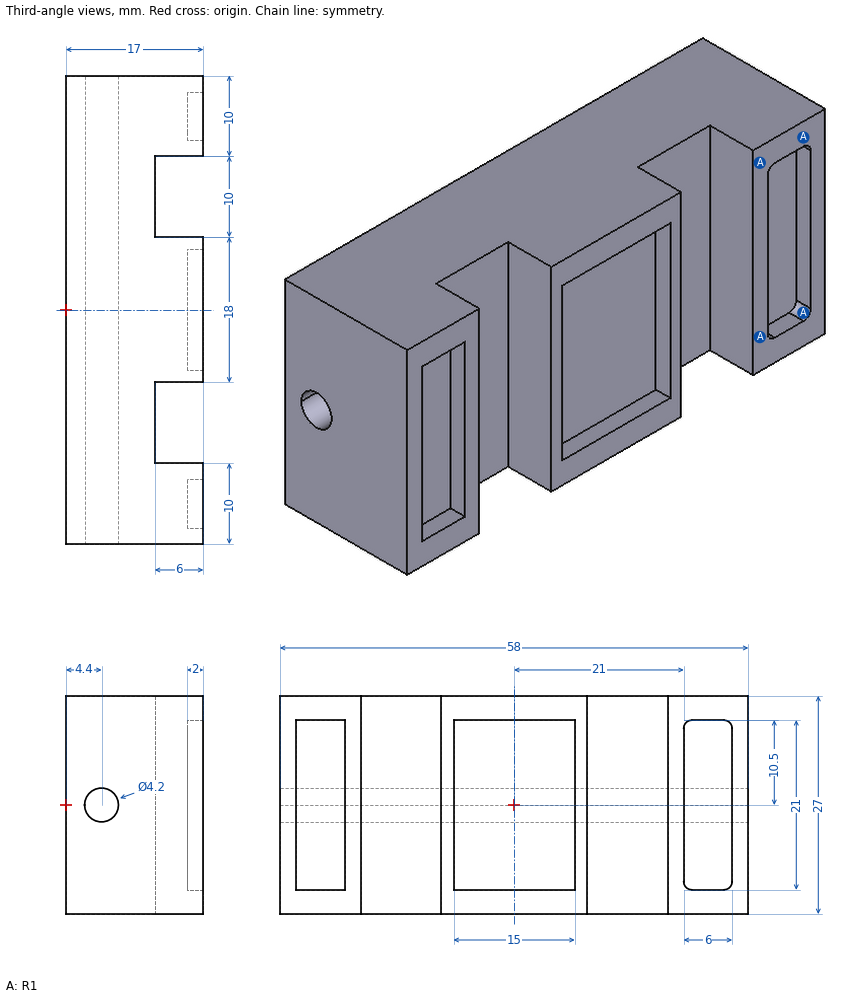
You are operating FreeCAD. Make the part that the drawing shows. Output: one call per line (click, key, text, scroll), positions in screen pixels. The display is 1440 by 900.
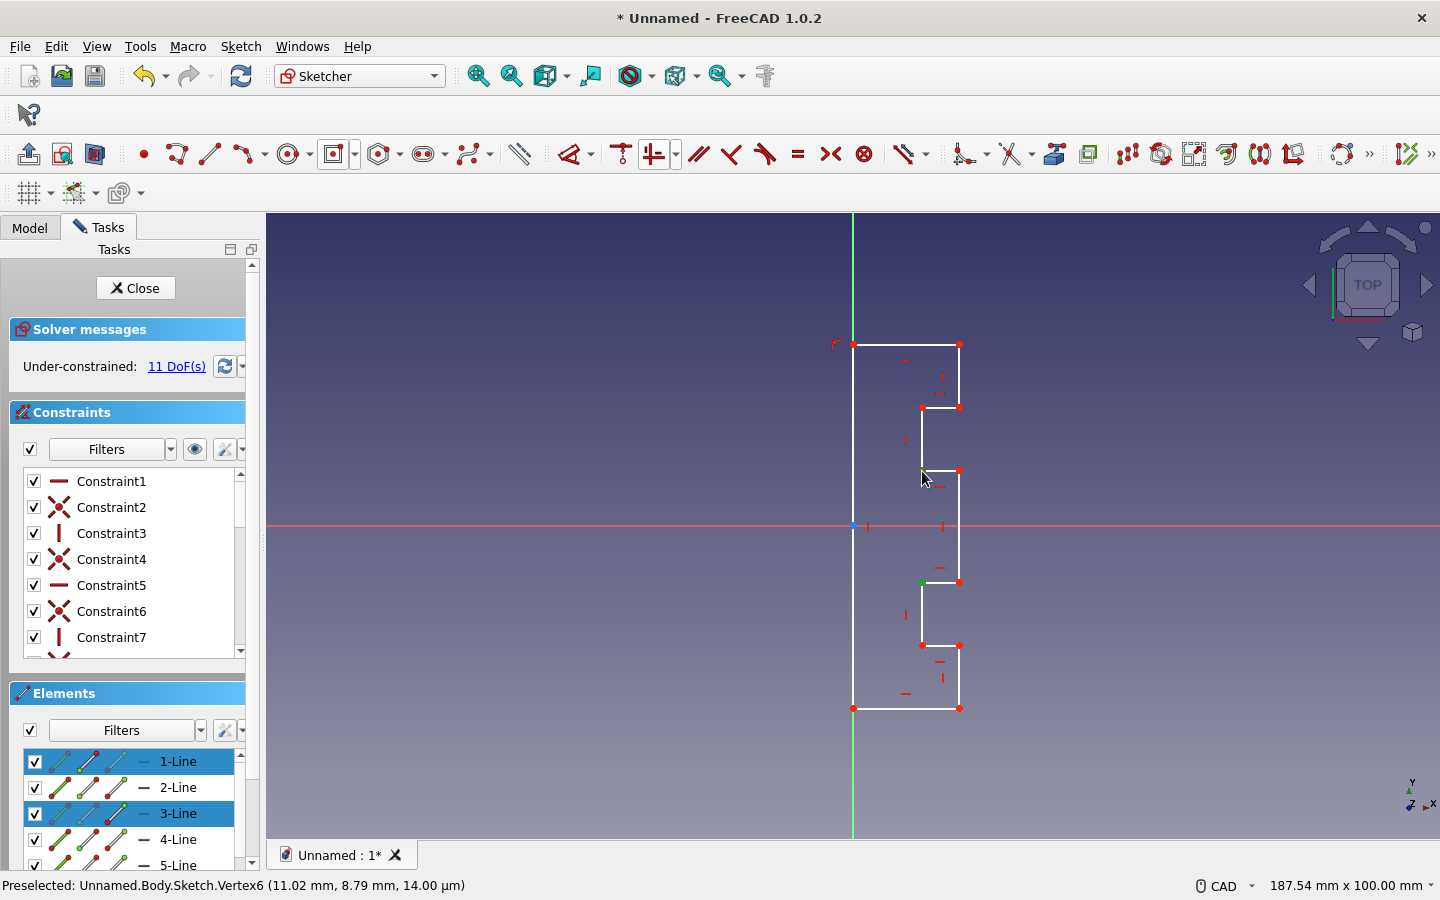
click(364, 526)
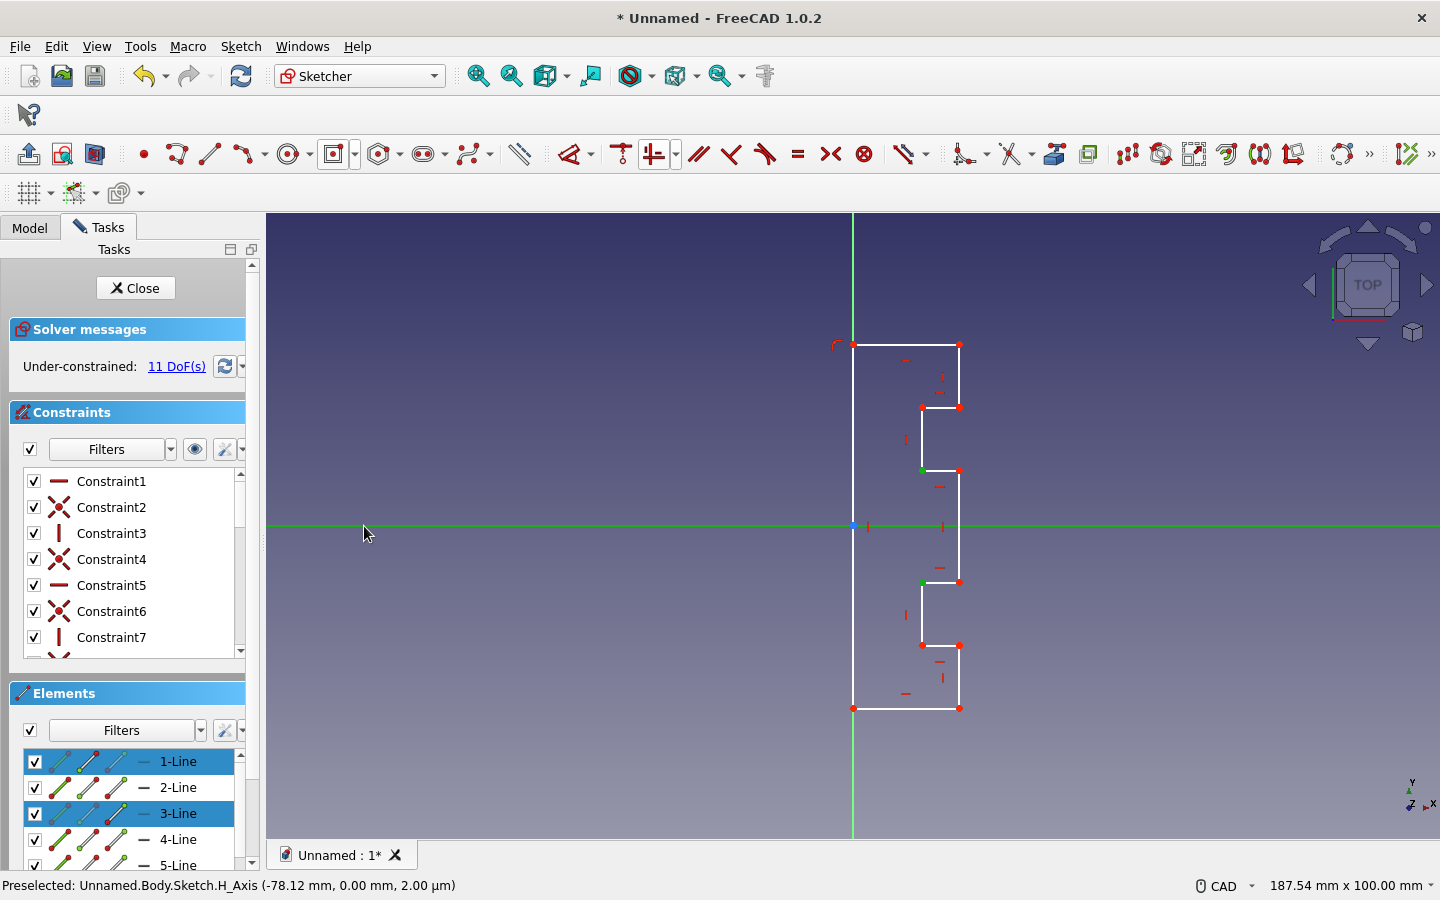
key(s)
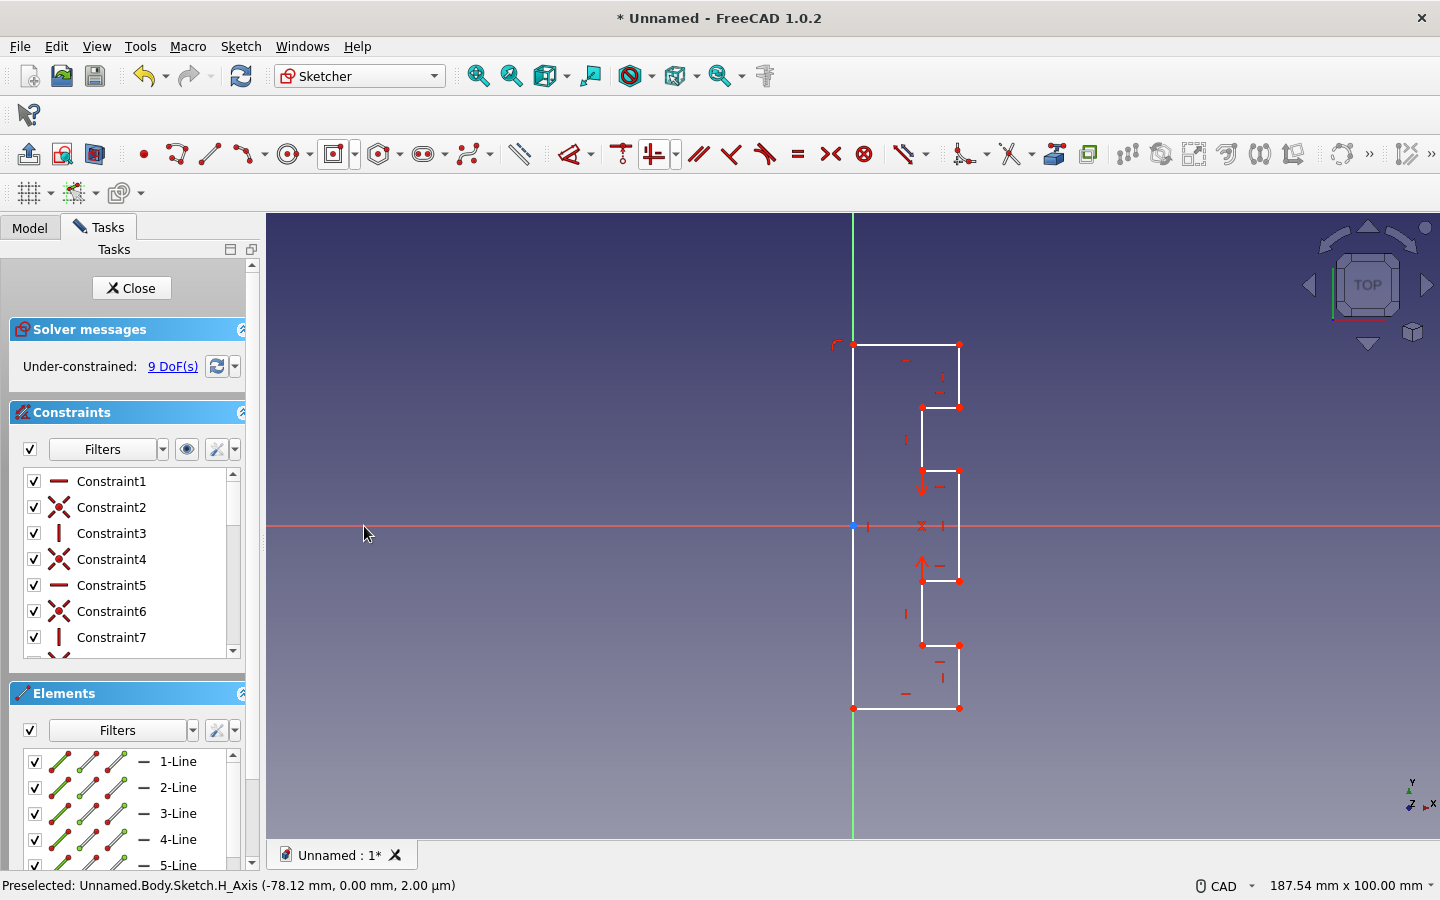
click(959, 345)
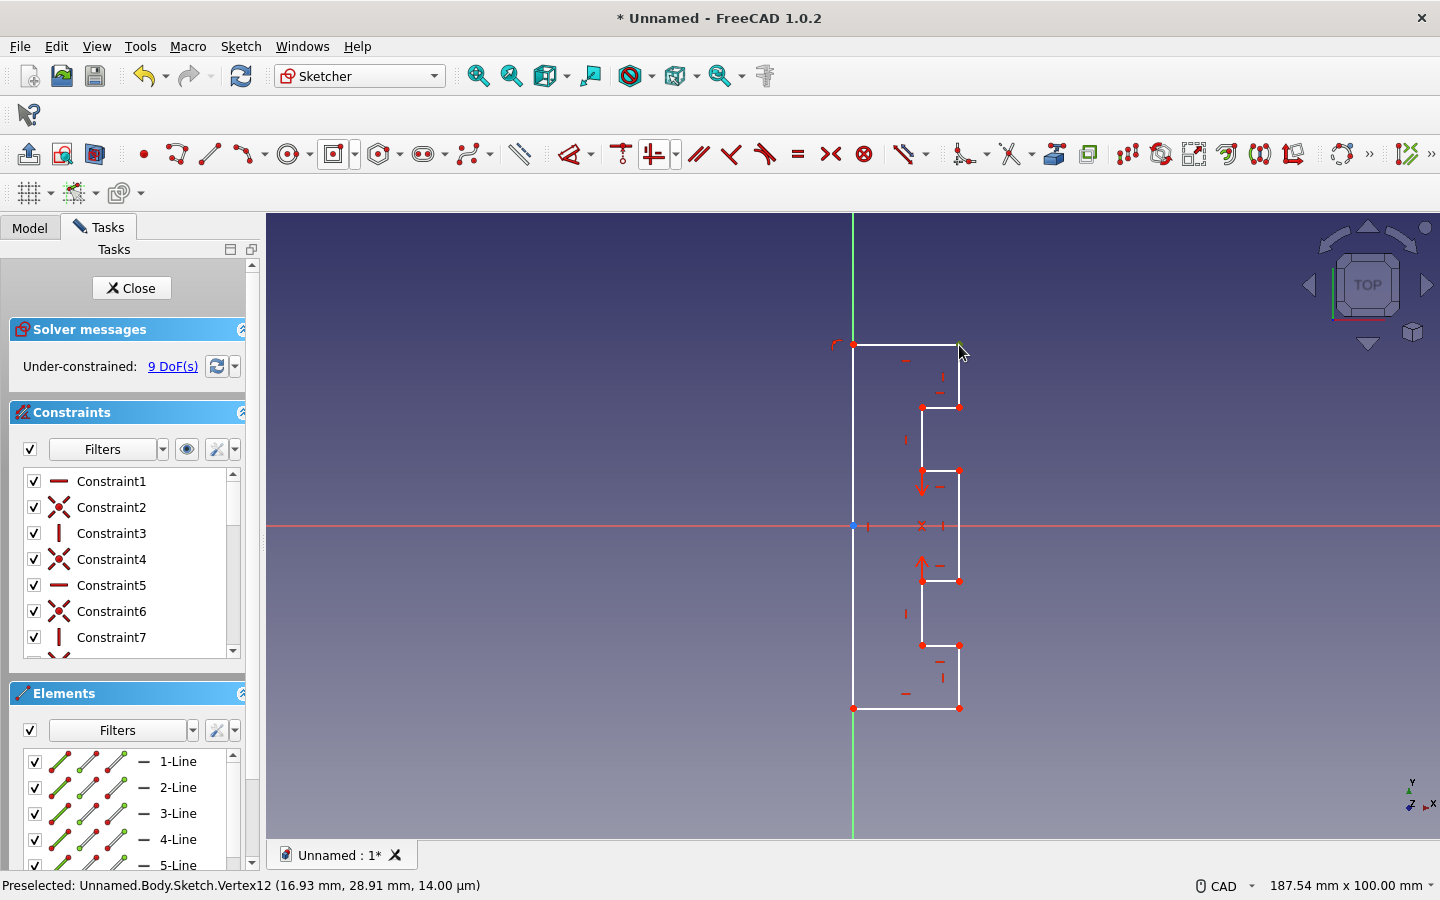
click(959, 709)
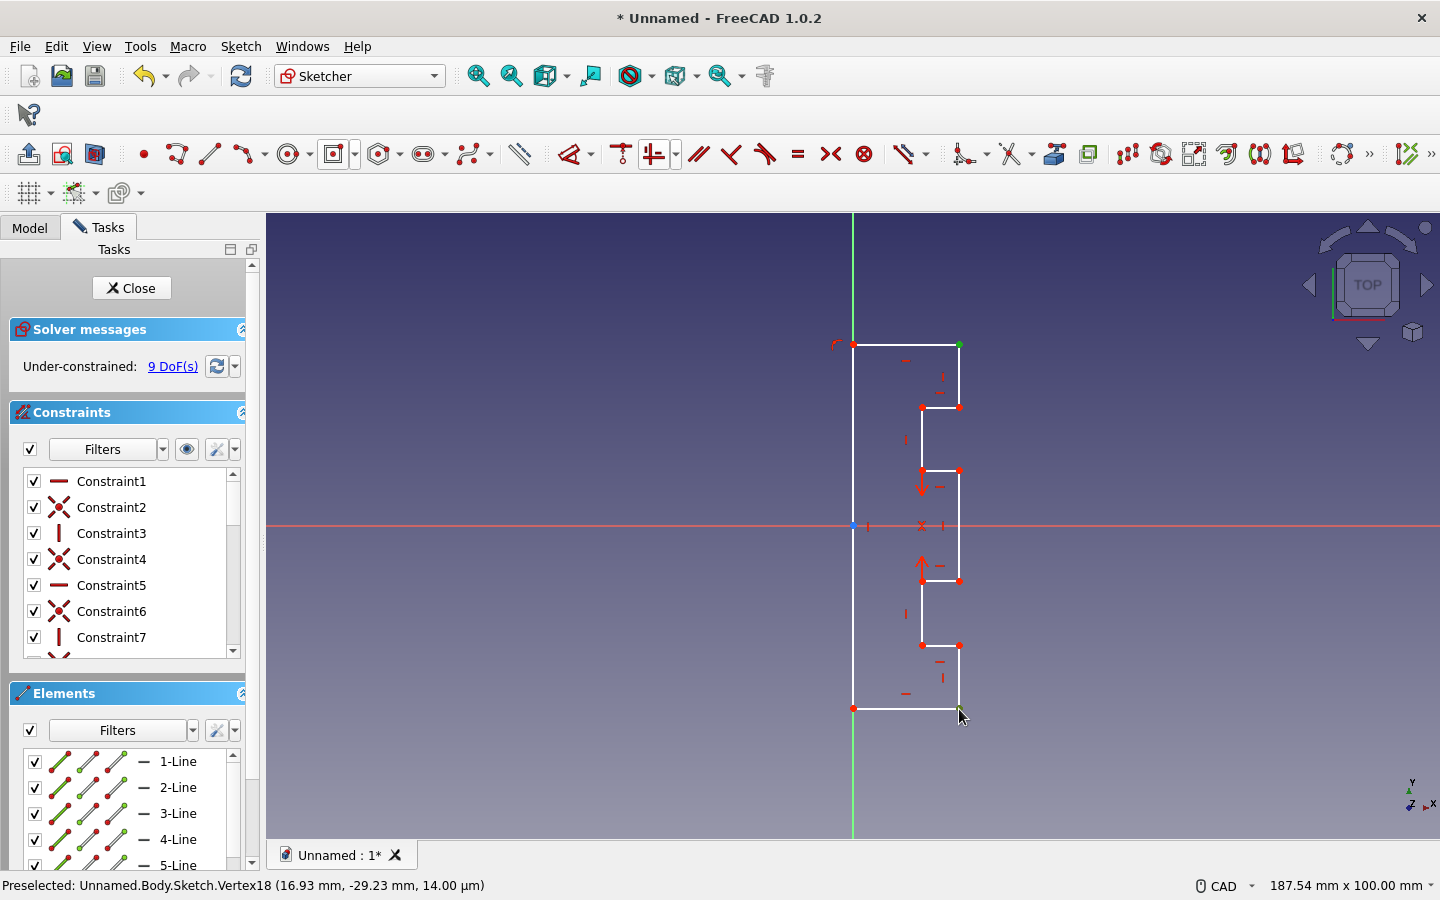
click(364, 526)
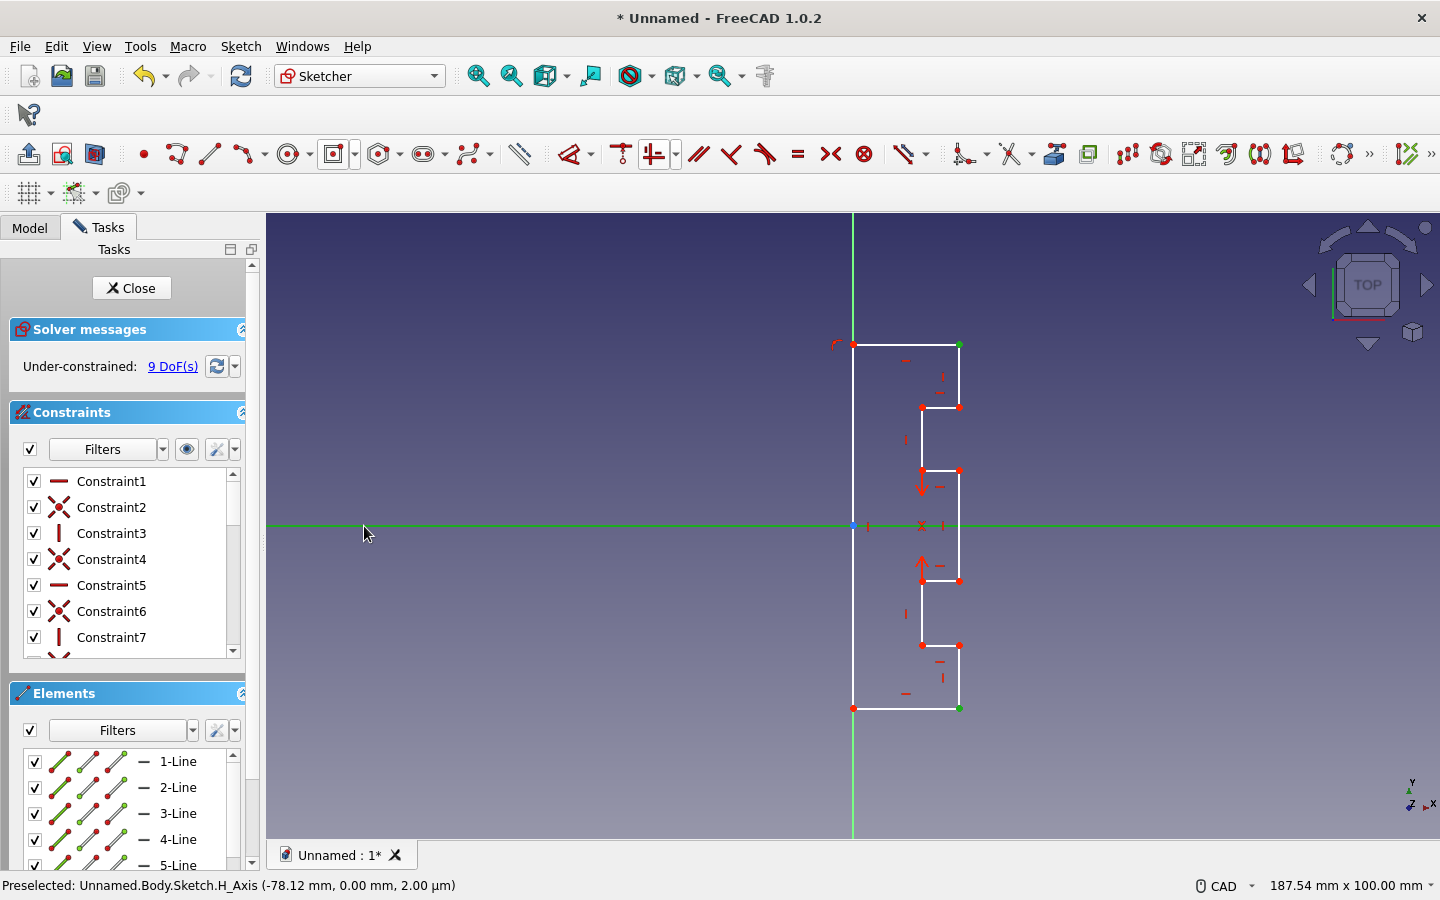
key(s)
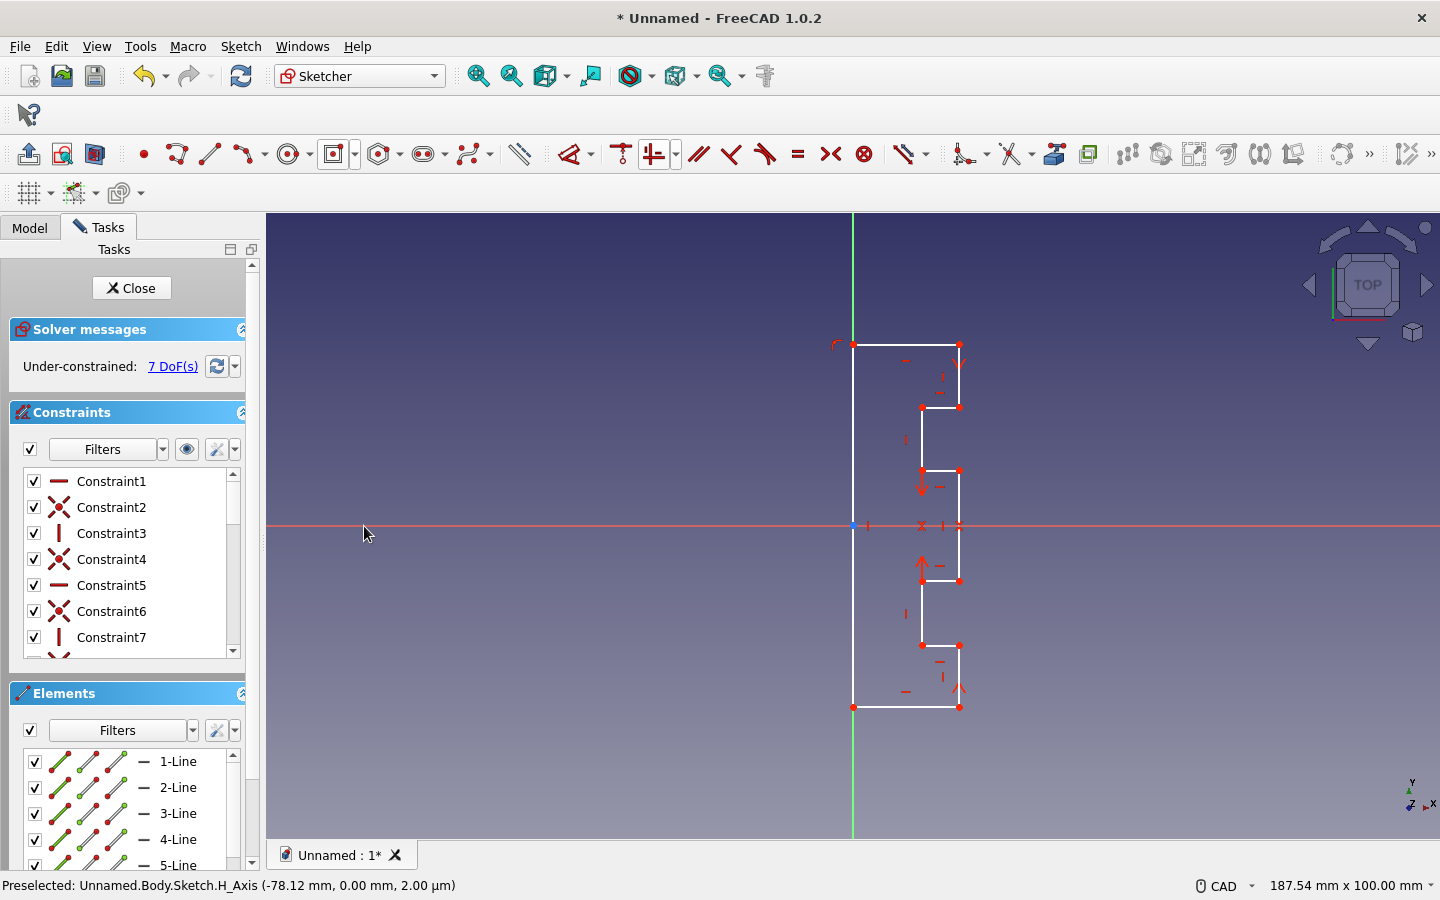
click(568, 154)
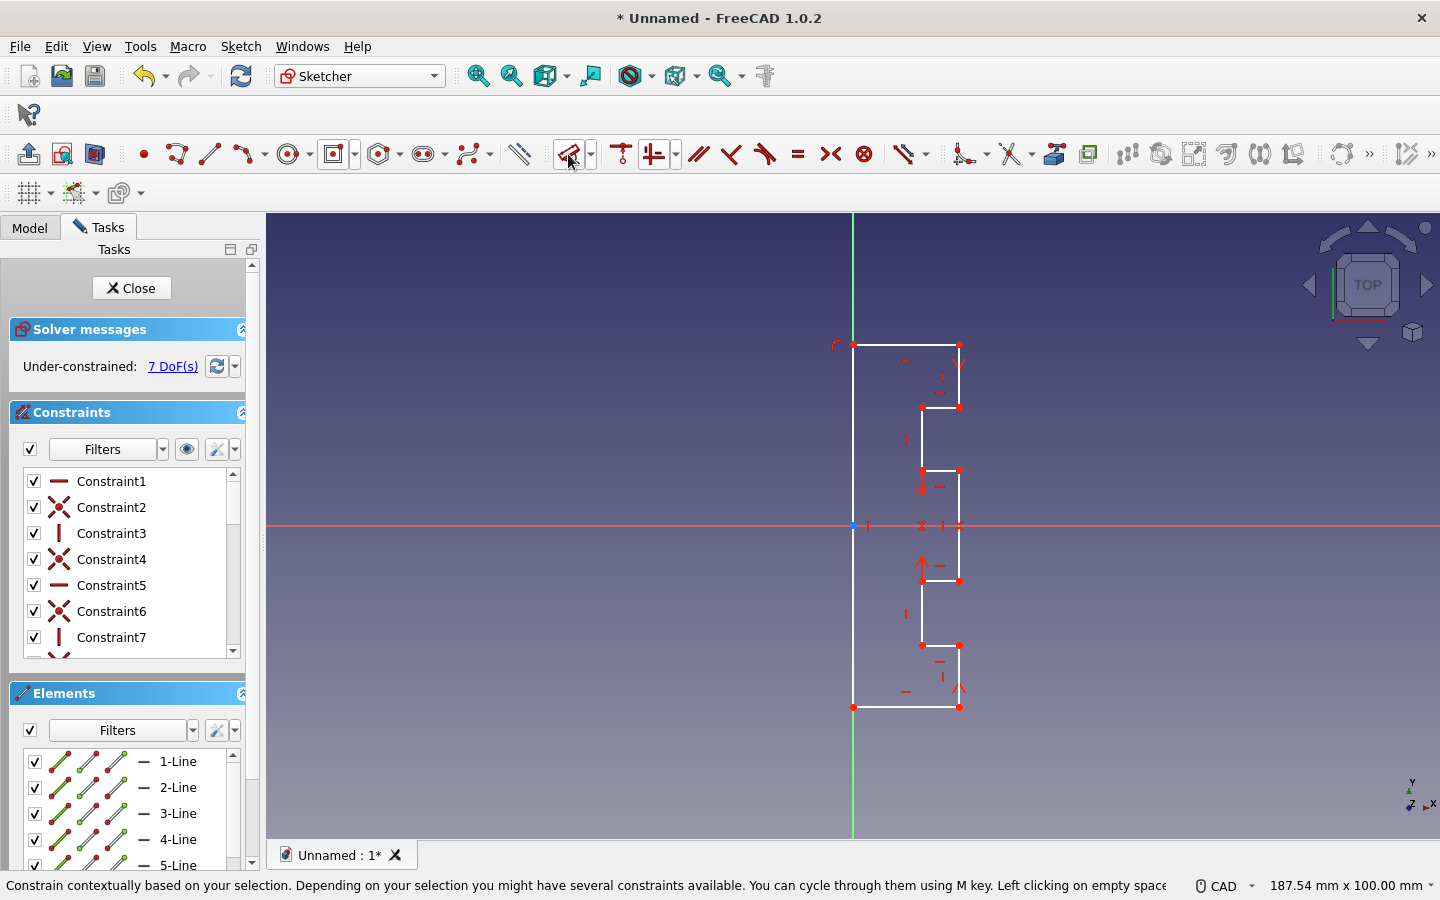
scroll(933, 581, up, 2)